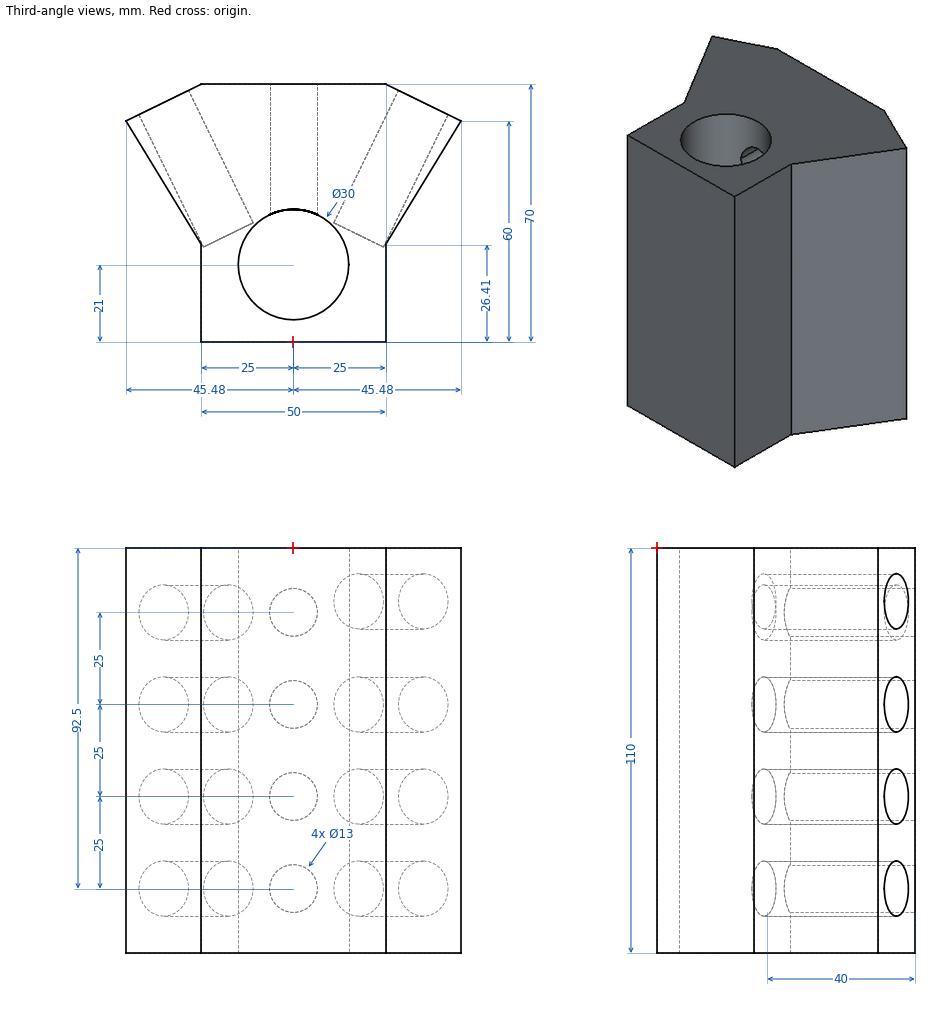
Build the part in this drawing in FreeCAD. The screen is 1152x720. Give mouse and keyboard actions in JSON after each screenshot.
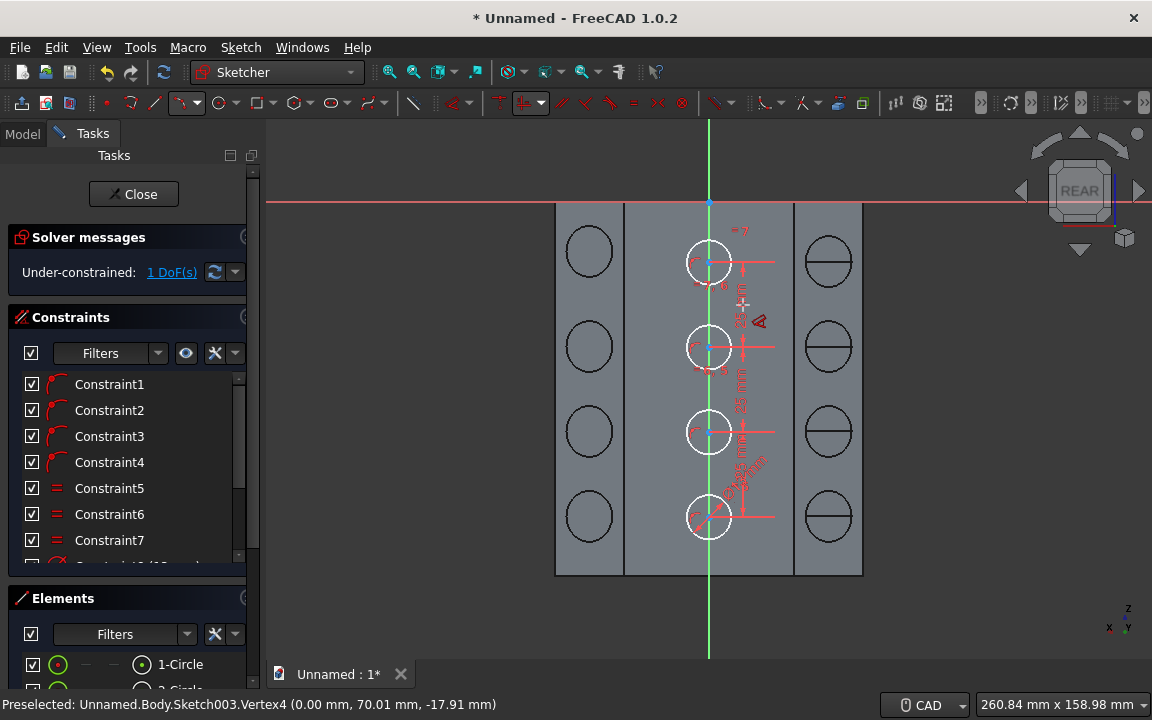
{"action": "left_click", "coordinate": [709, 517]}
{"action": "left_click", "coordinate": [743, 360]}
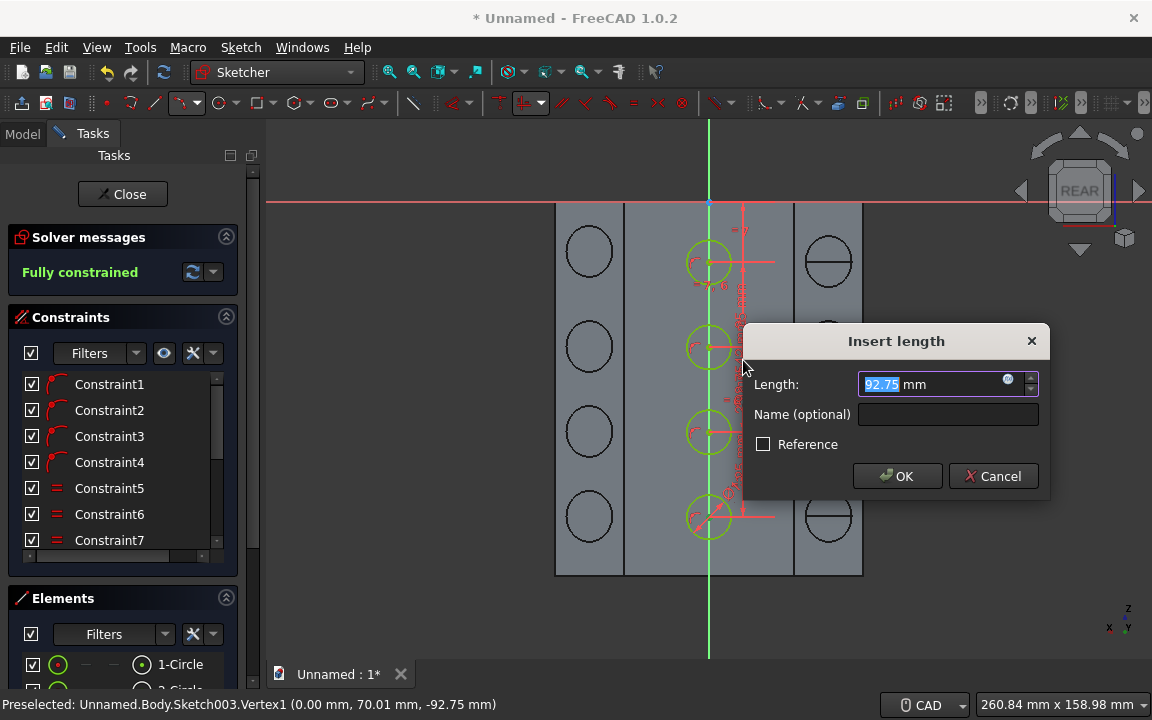
{"action": "type", "text": "92.5"}
{"action": "key", "text": "Return"}
{"action": "key", "text": "Escape"}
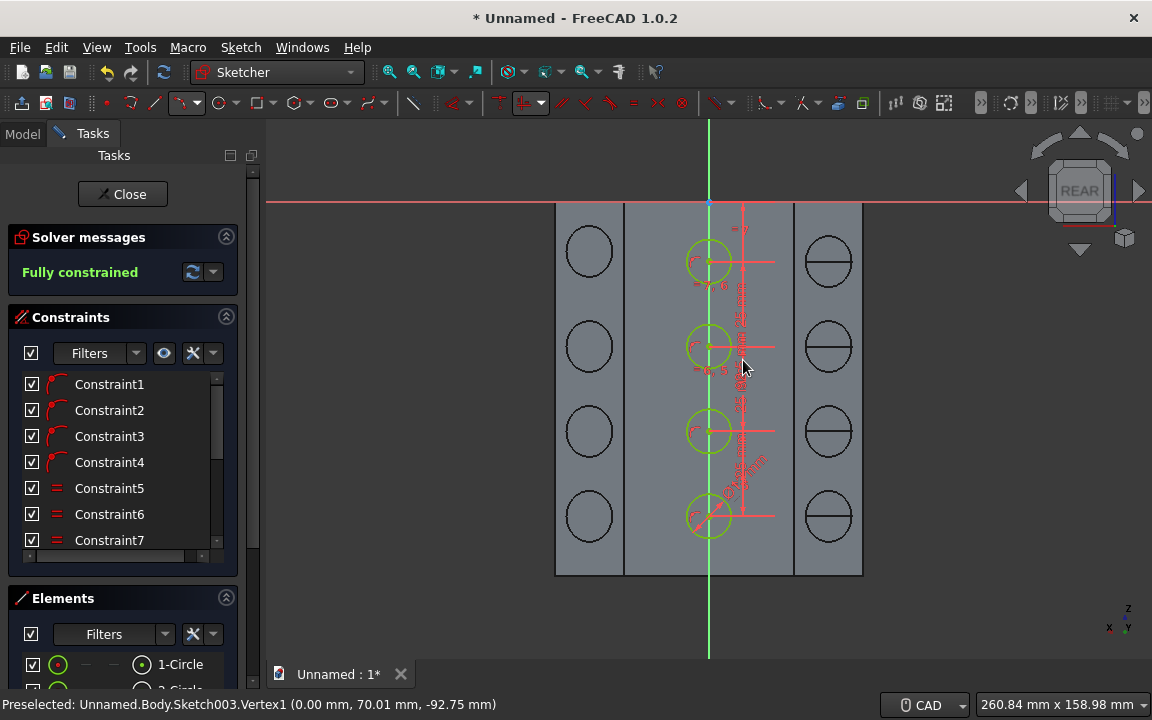
{"action": "left_click", "coordinate": [123, 194]}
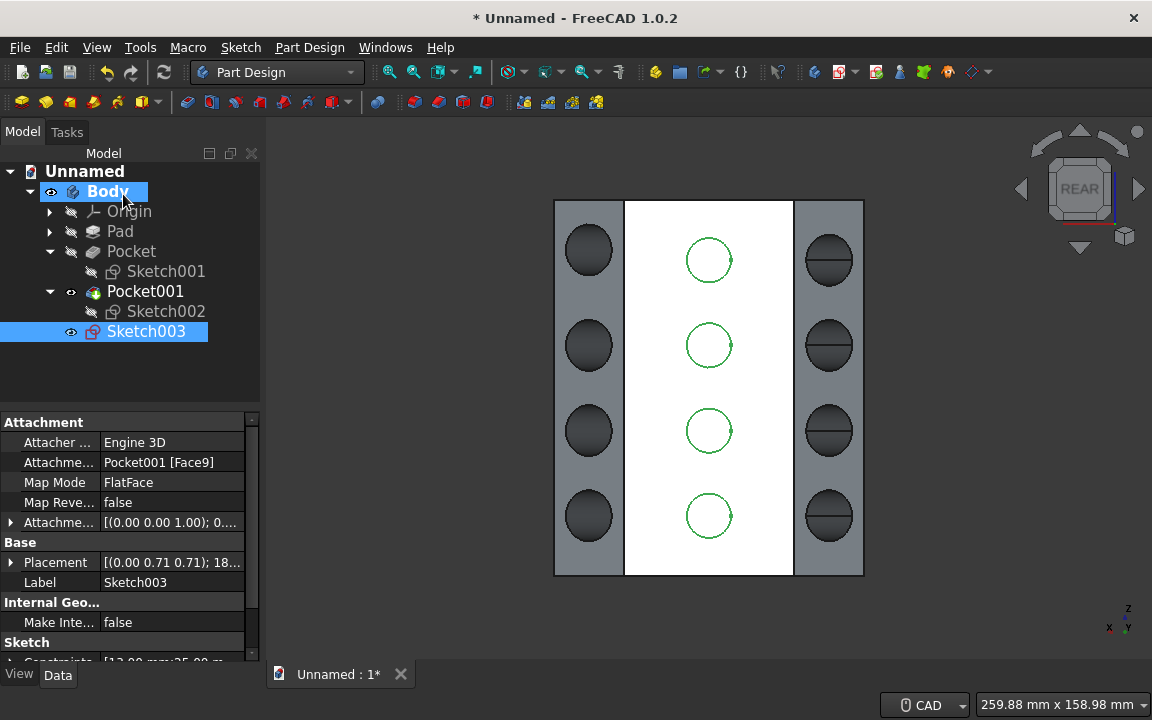
{"action": "left_click", "coordinate": [188, 102]}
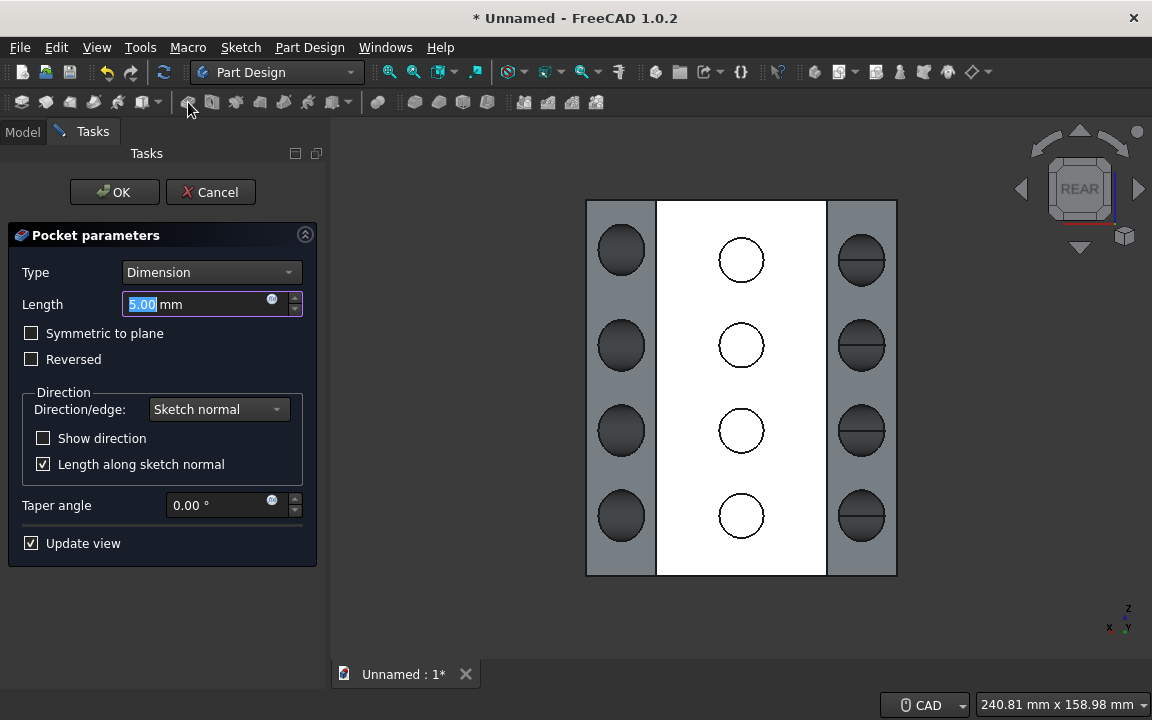
{"action": "type", "text": "40"}
{"action": "key", "text": "Tab"}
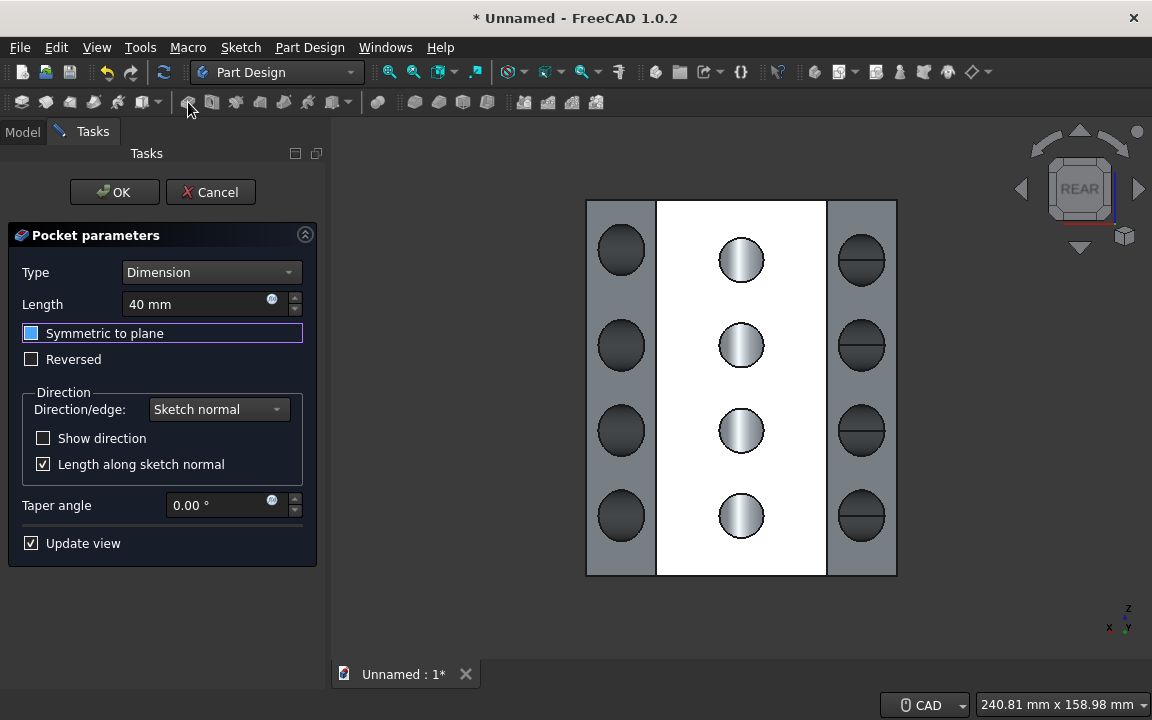
{"action": "left_click", "coordinate": [115, 192]}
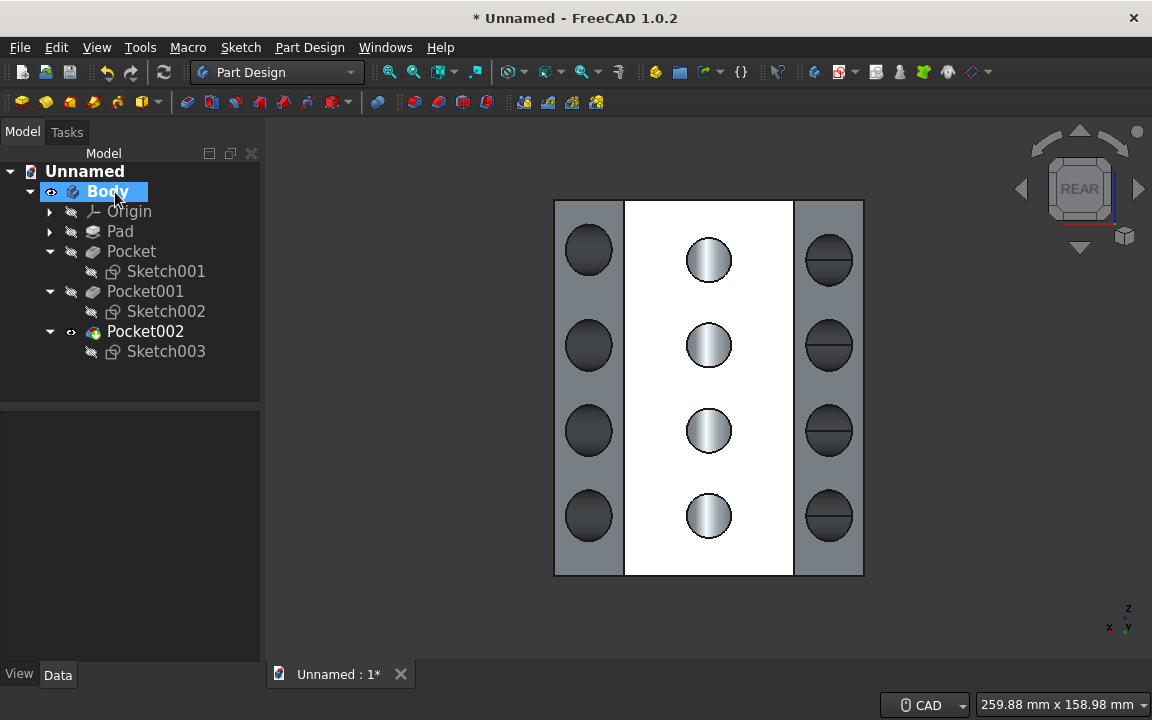
{"action": "key", "text": "0"}